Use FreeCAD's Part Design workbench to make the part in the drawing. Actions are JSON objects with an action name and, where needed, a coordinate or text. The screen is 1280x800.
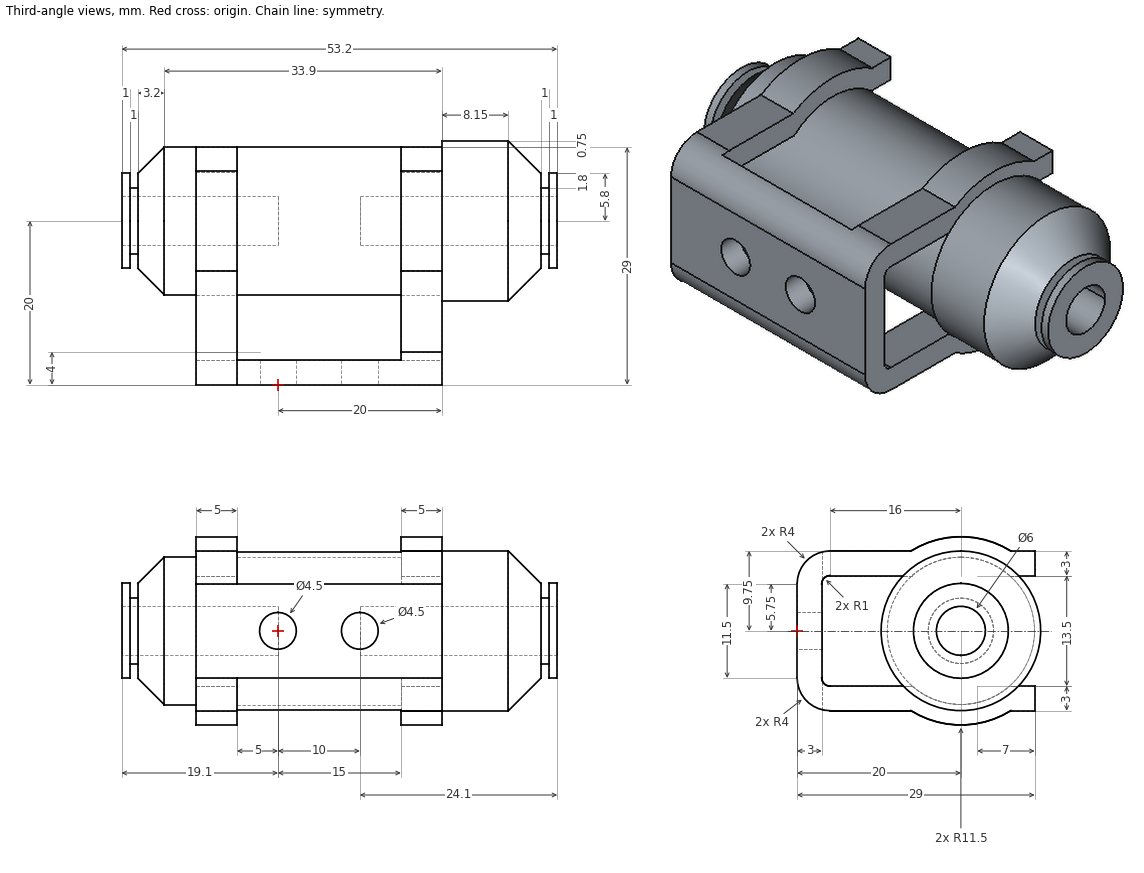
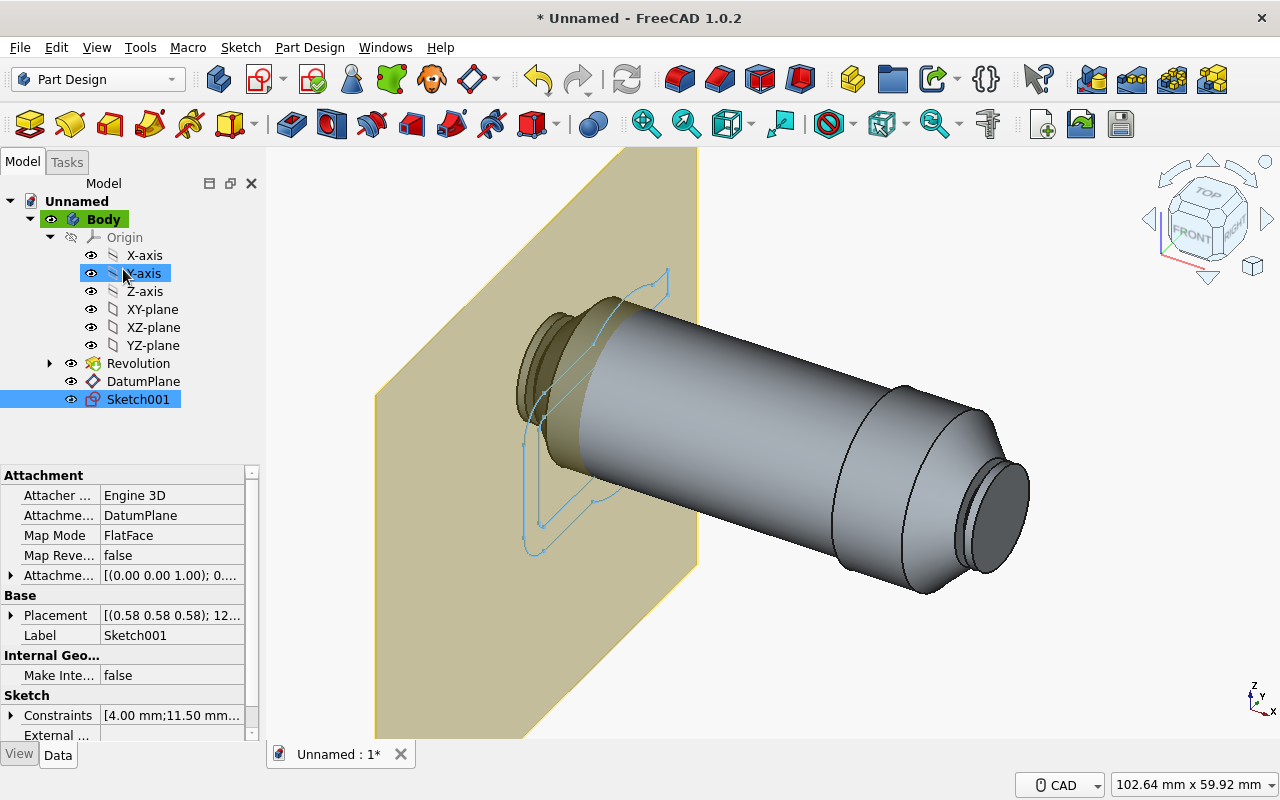
{"action": "left_click", "coordinate": [30, 124]}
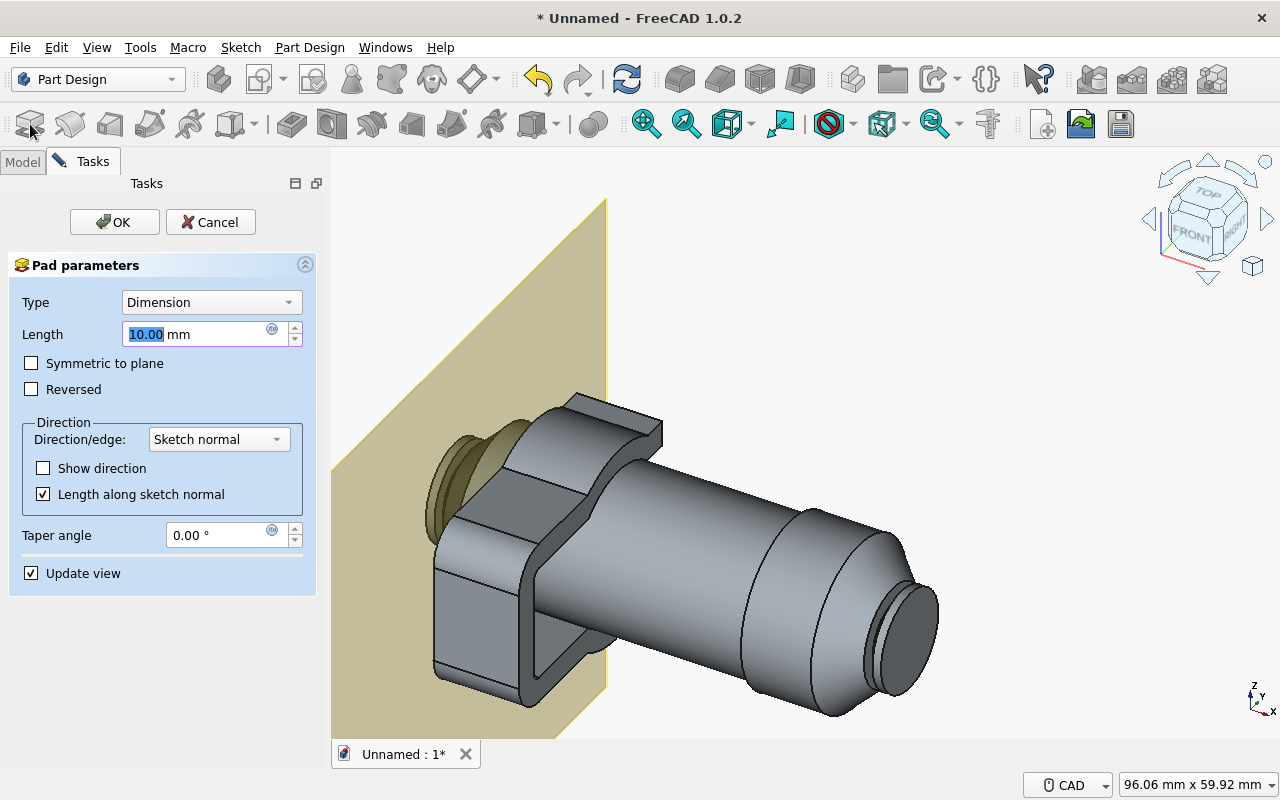
{"action": "type", "text": "5"}
{"action": "key", "text": "Tab"}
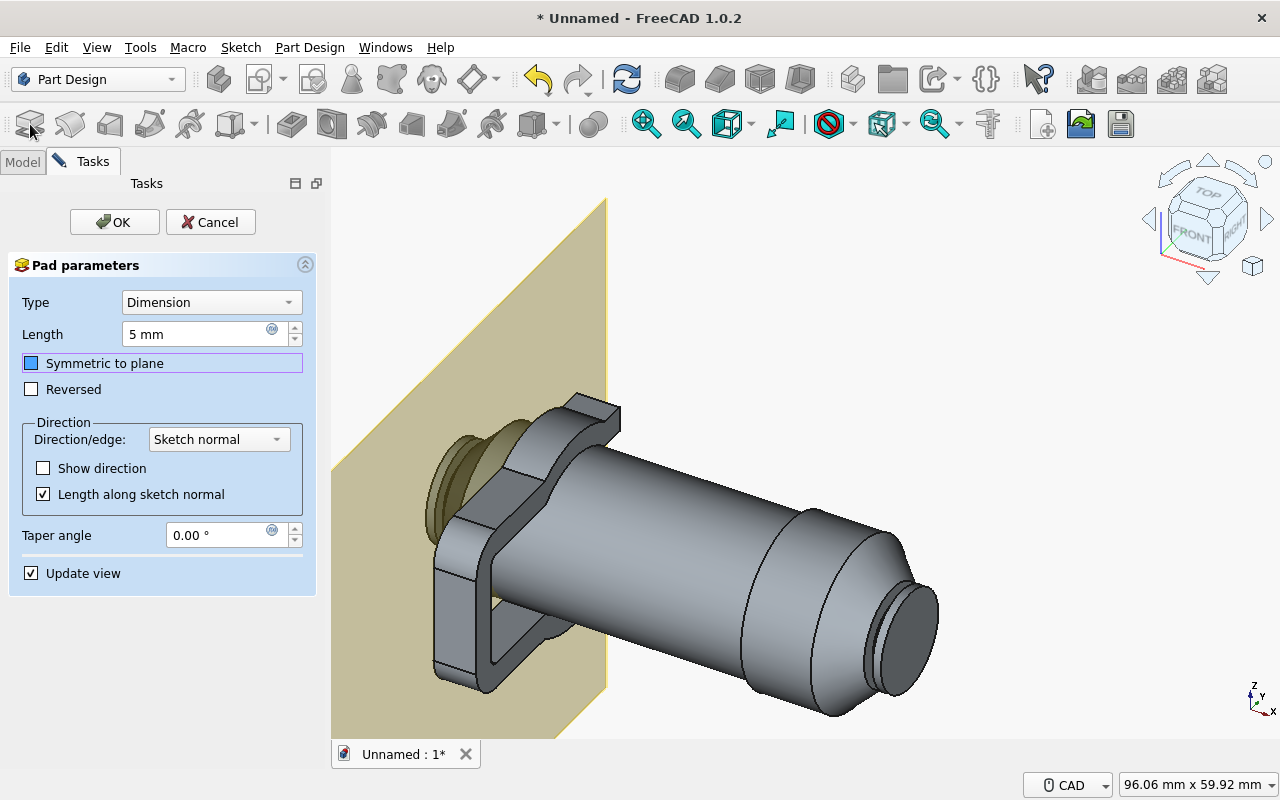
{"action": "left_click", "coordinate": [115, 222]}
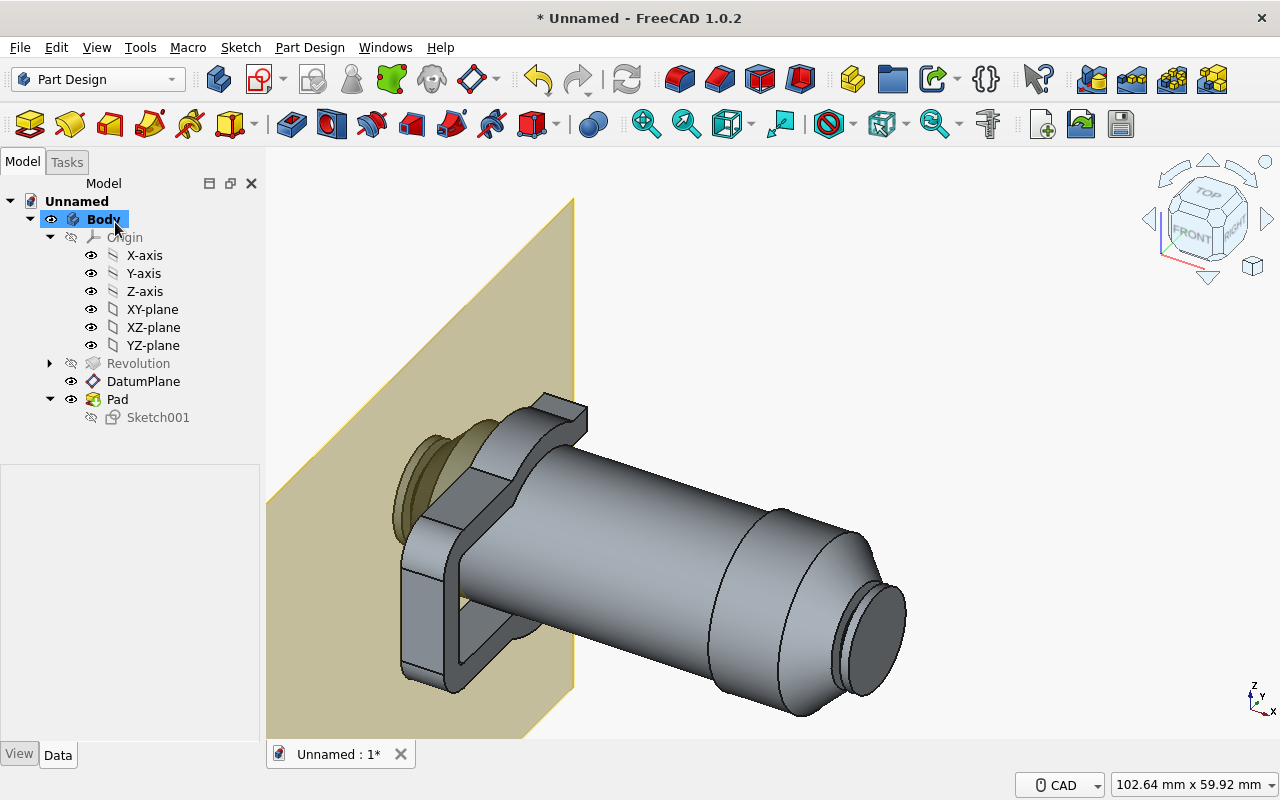
{"action": "left_click", "coordinate": [116, 381]}
{"action": "key", "text": "space"}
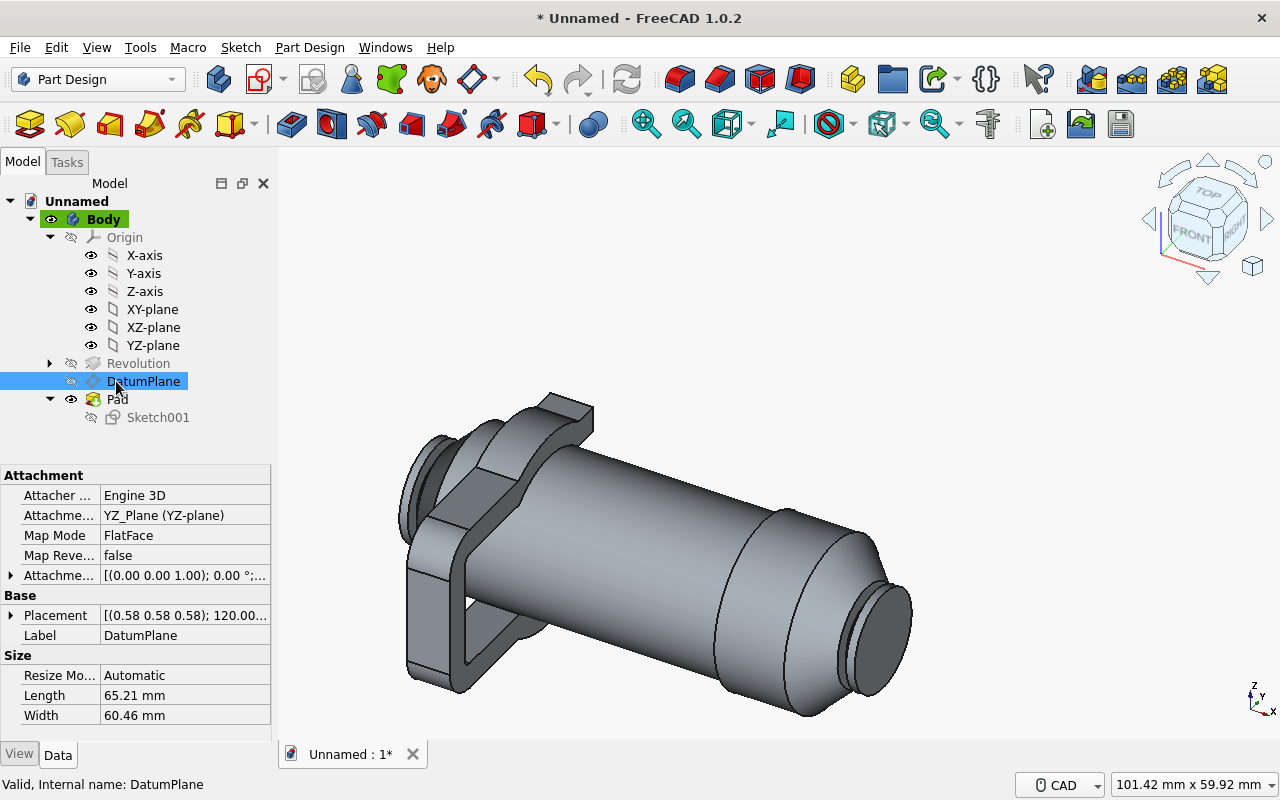
{"action": "left_click", "coordinate": [648, 124]}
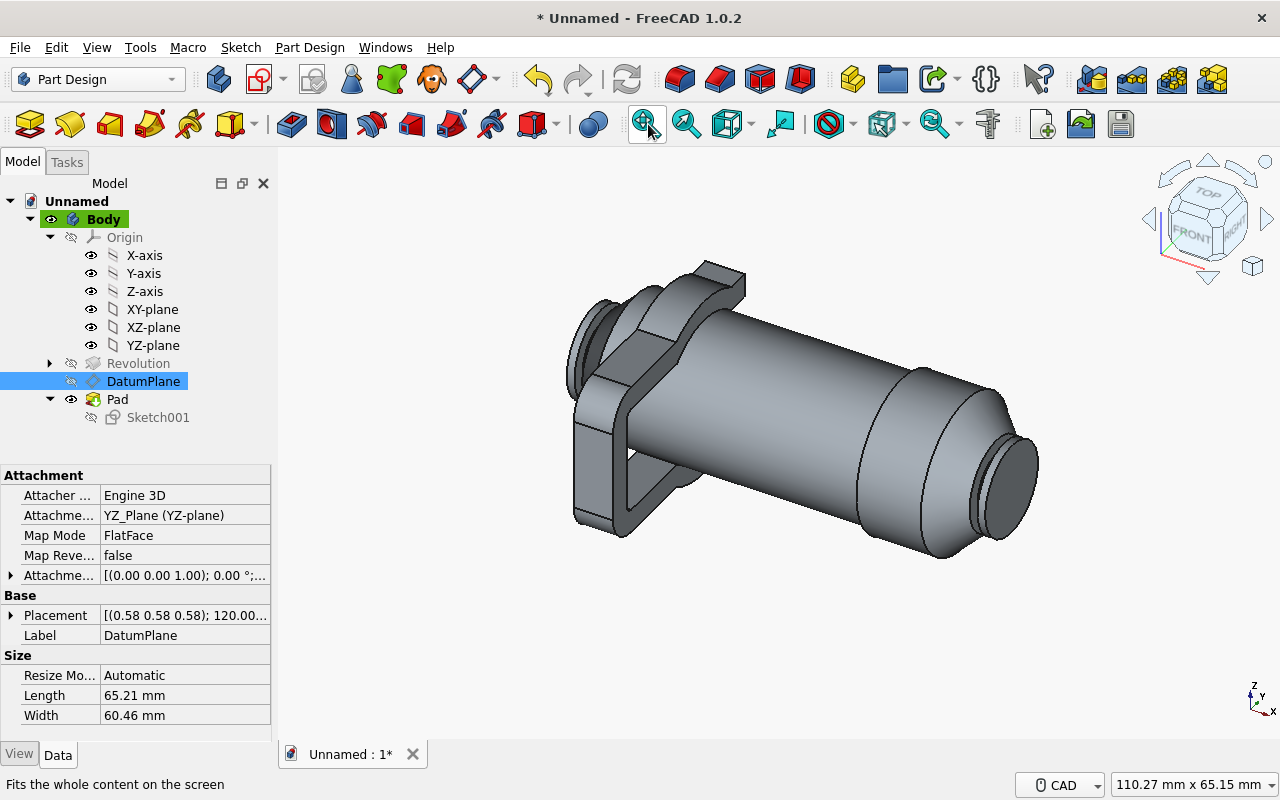
{"action": "left_click", "coordinate": [136, 345]}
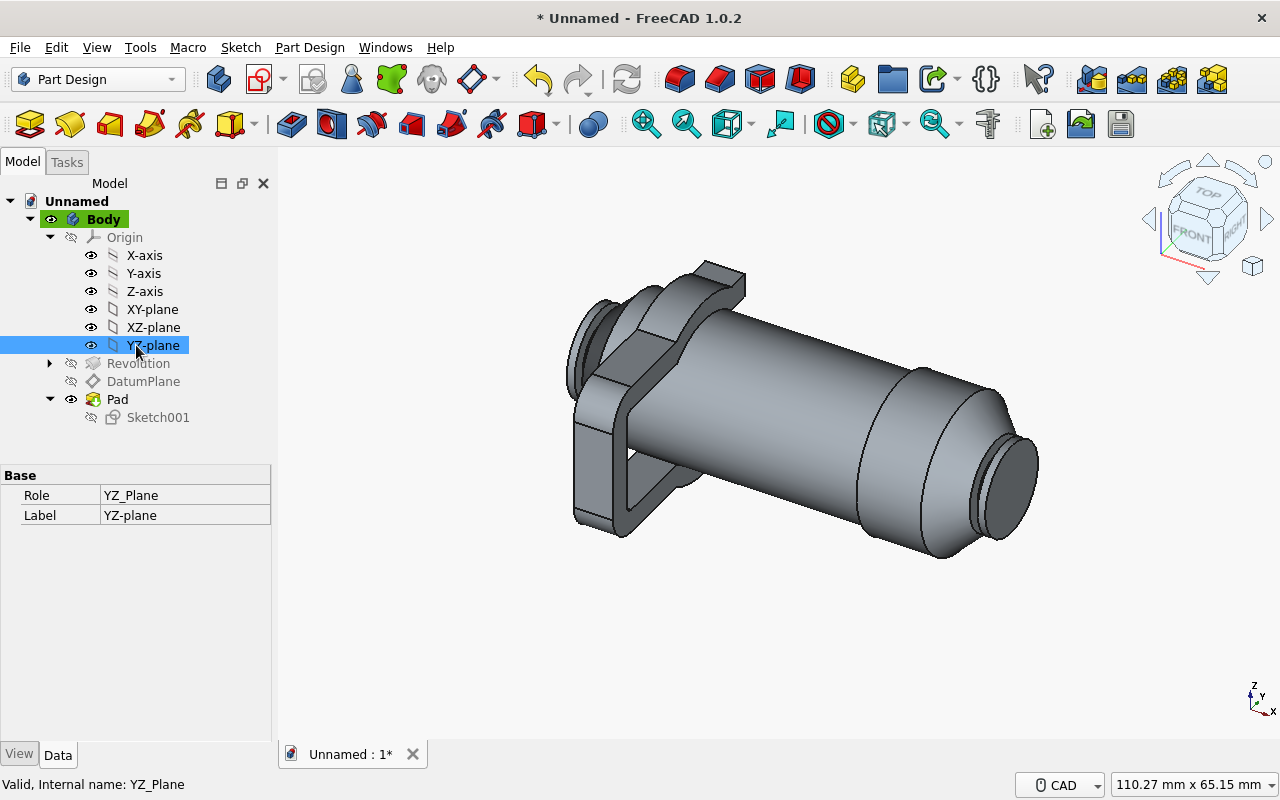
{"action": "left_click", "coordinate": [472, 80]}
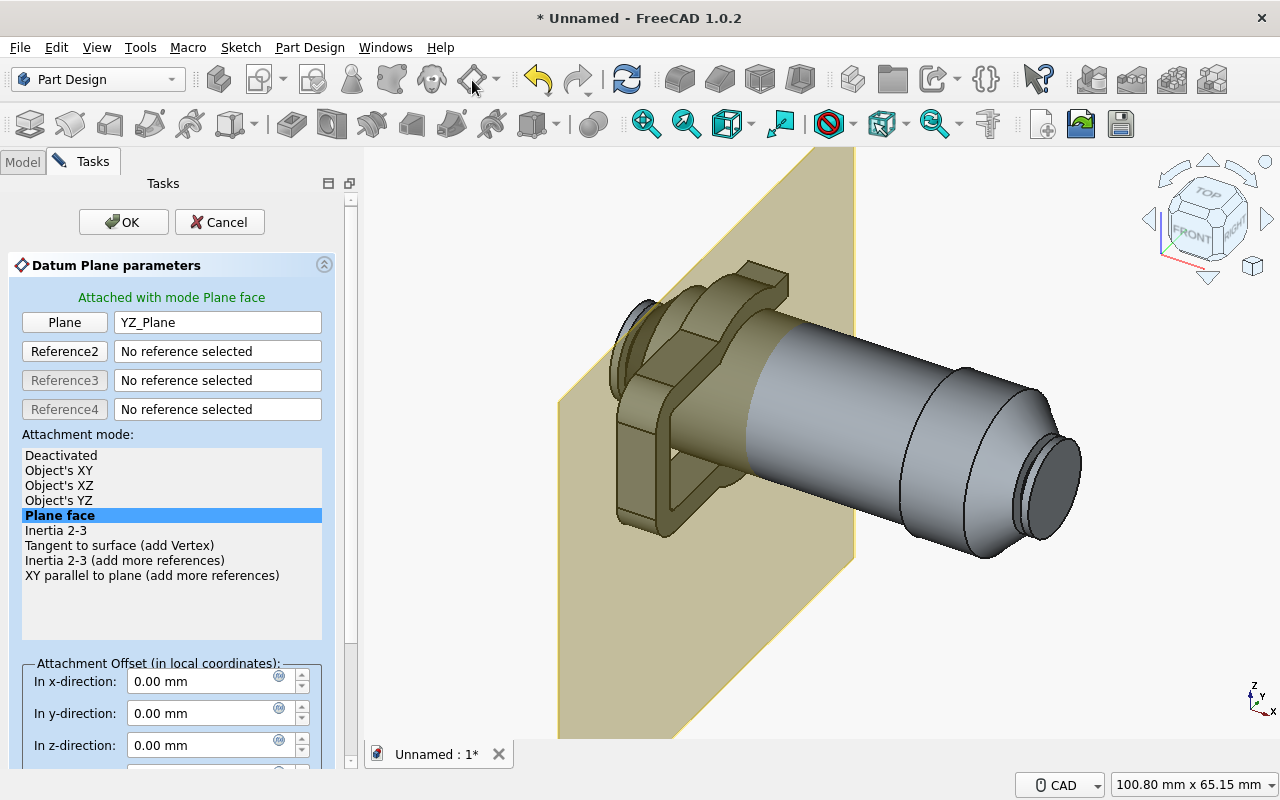
{"action": "triple_click", "coordinate": [210, 745]}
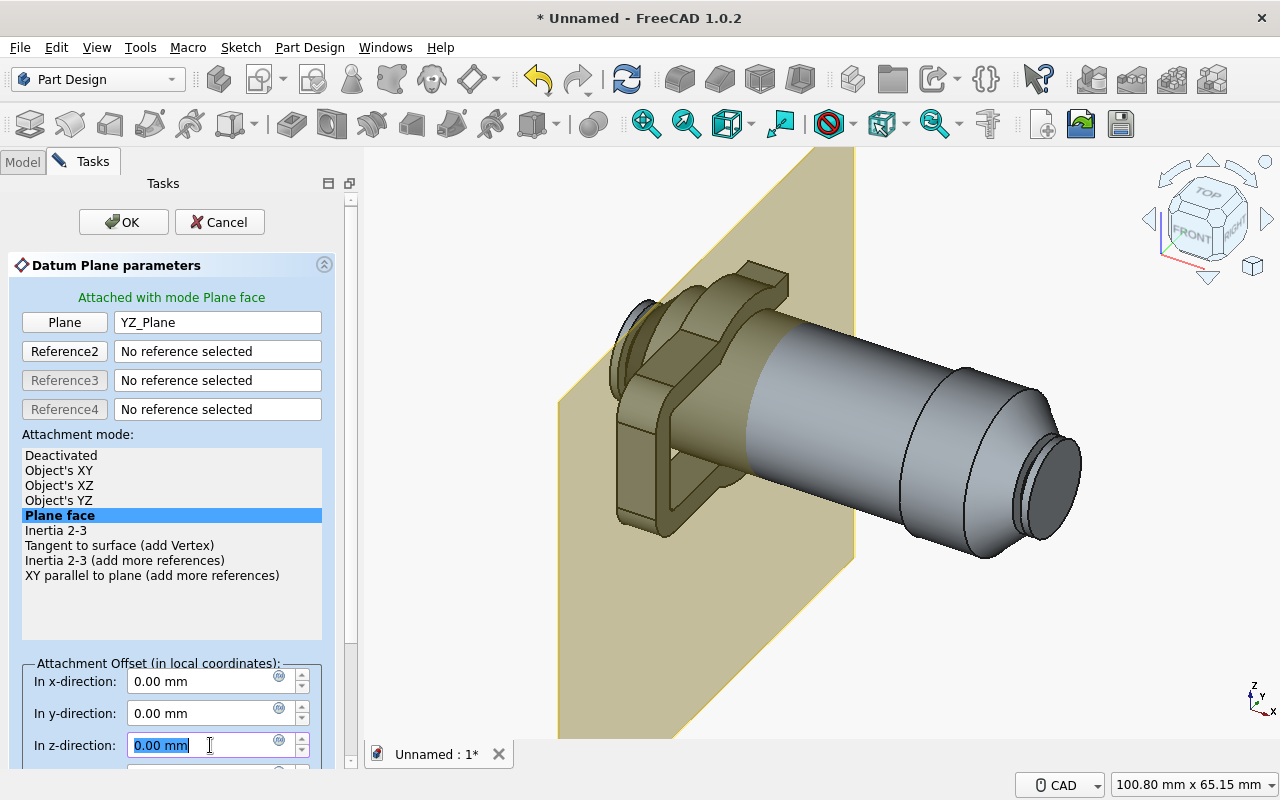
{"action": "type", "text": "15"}
{"action": "key", "text": "Tab"}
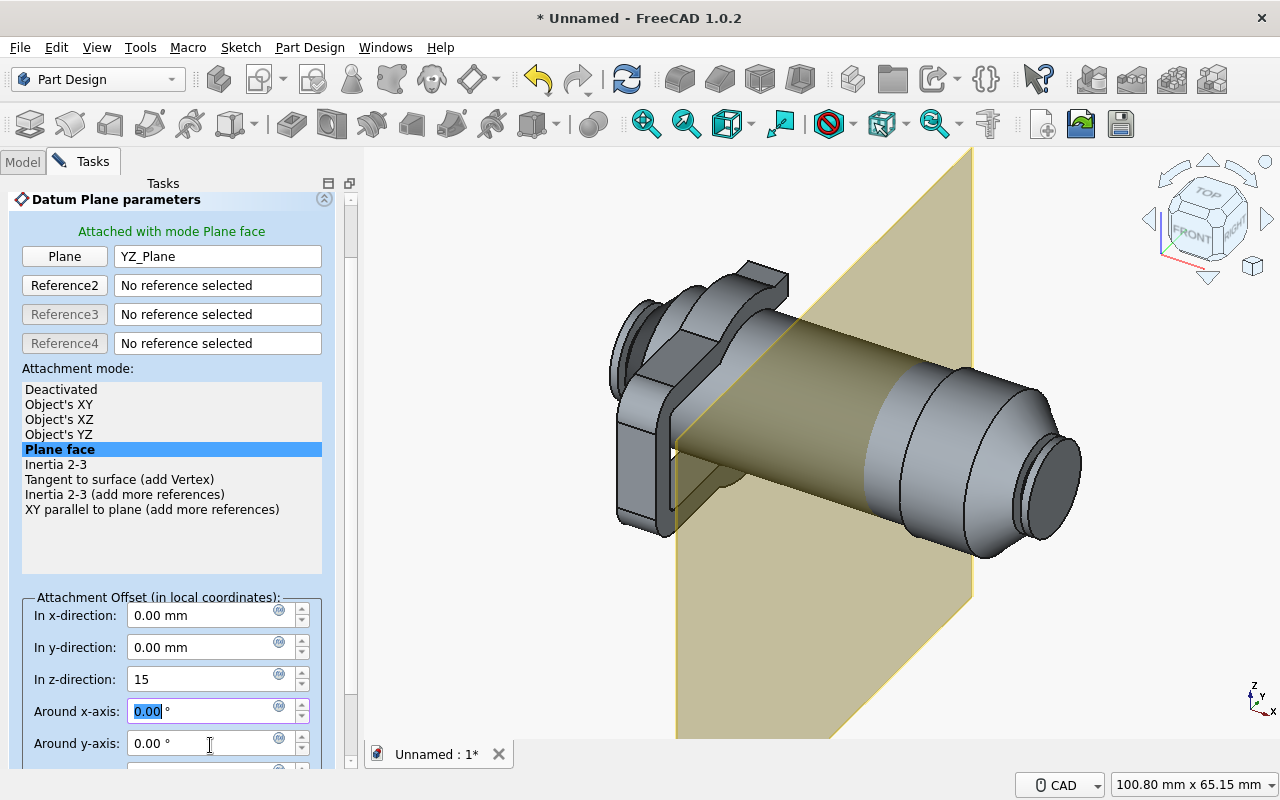
{"action": "scroll", "coordinate": [351, 480], "scroll_direction": "up", "scroll_amount": 2}